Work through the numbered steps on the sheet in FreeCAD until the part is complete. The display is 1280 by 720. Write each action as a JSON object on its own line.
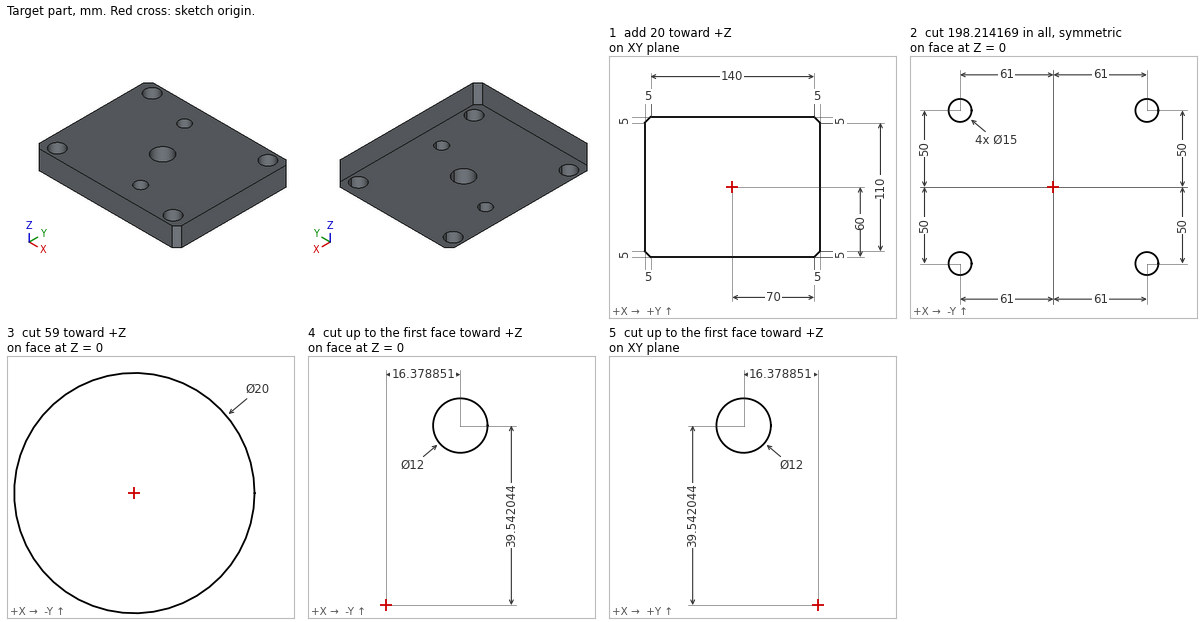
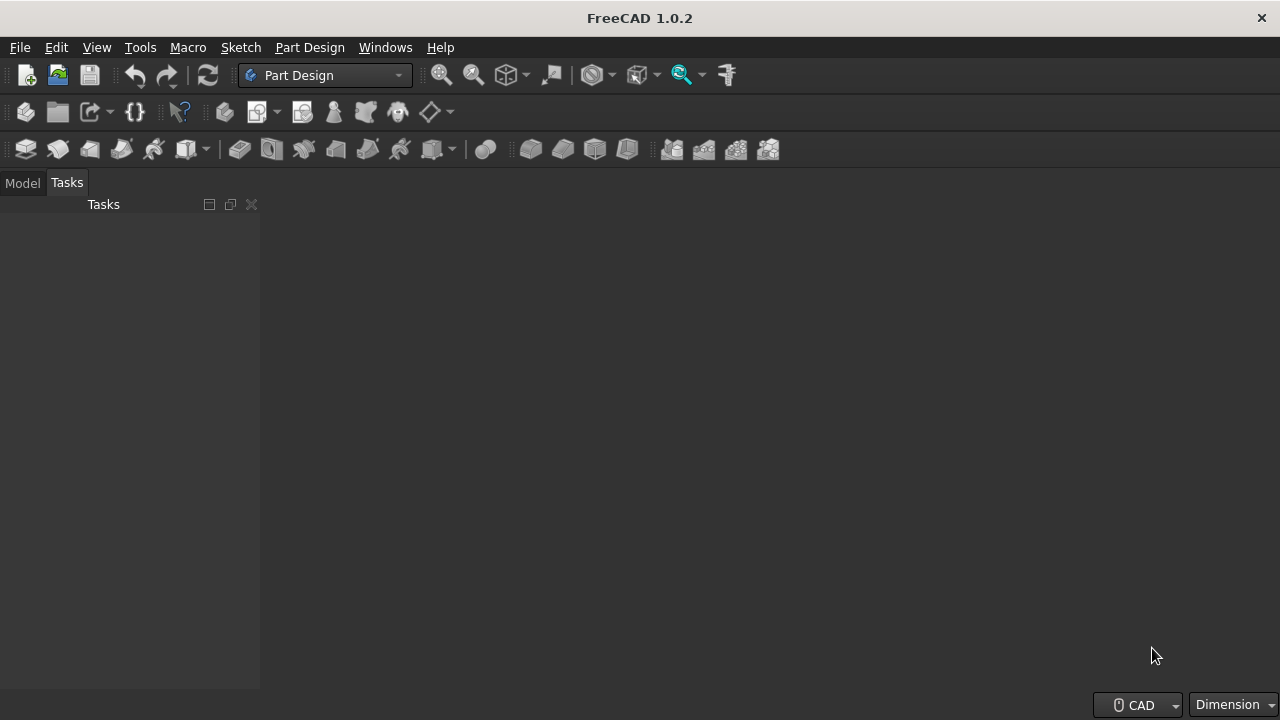
{"action": "key", "text": "ctrl+n"}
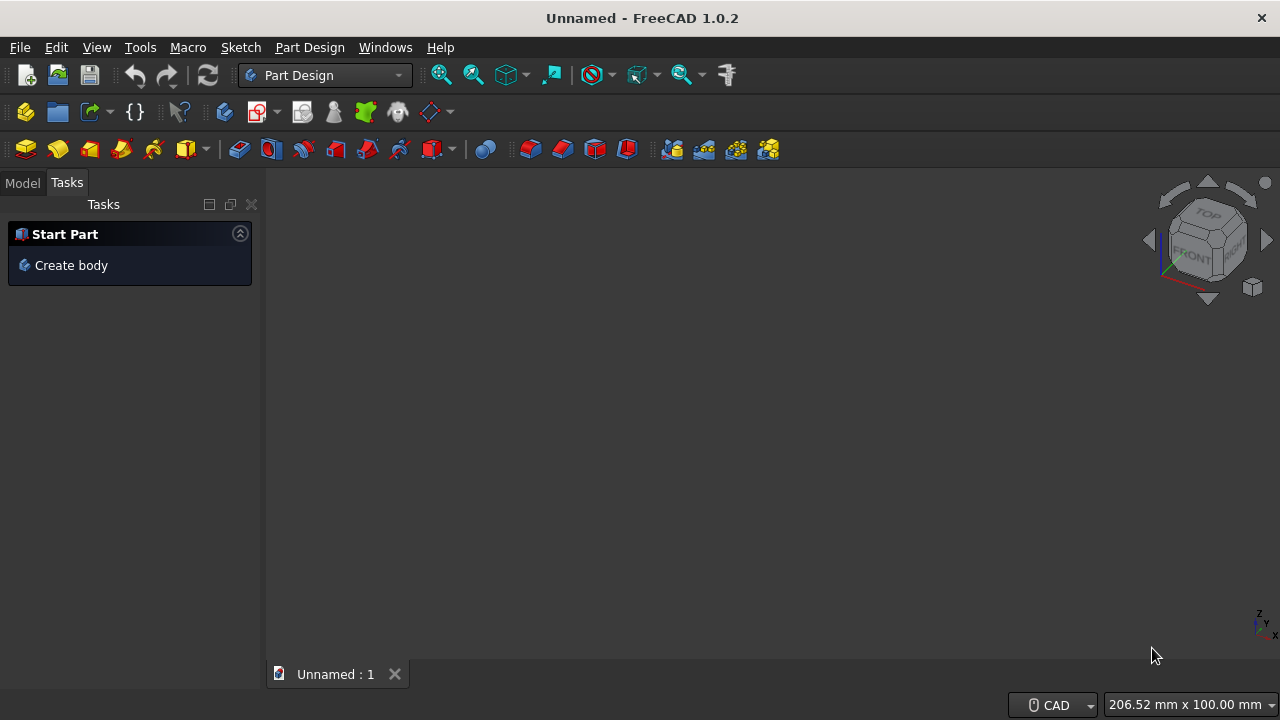
{"action": "left_click", "coordinate": [258, 112]}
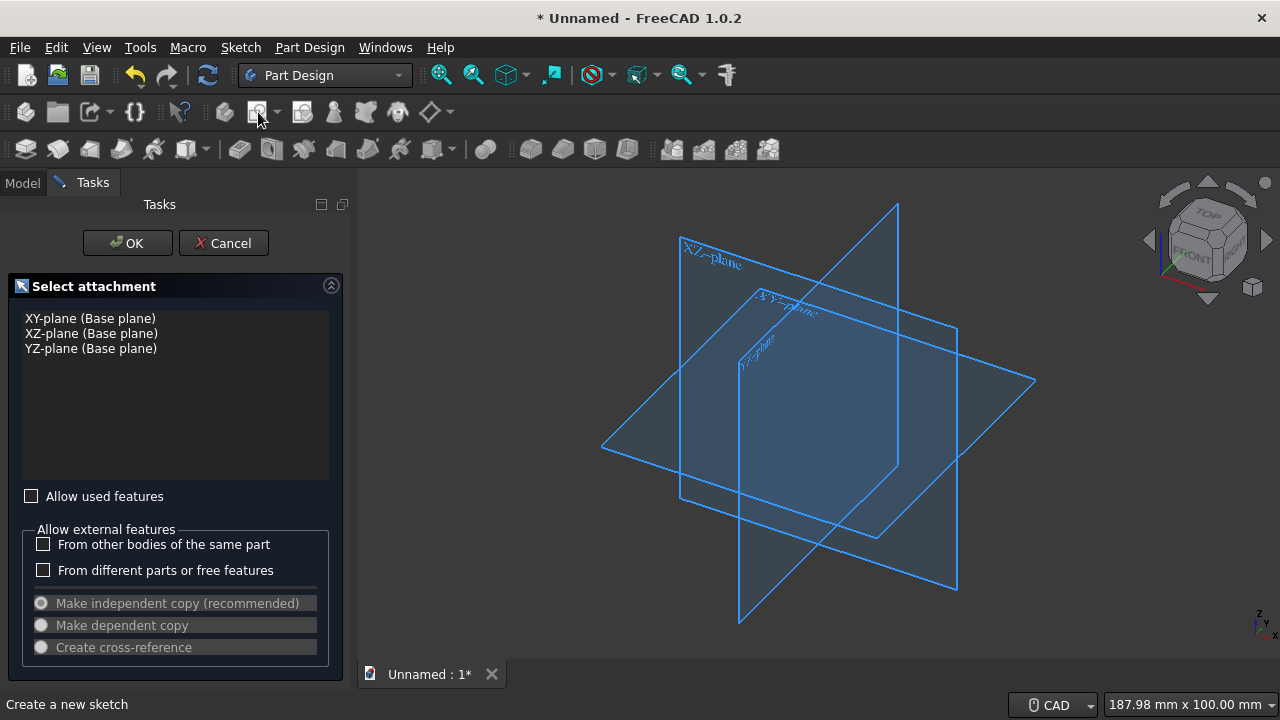
{"action": "left_click", "coordinate": [82, 318]}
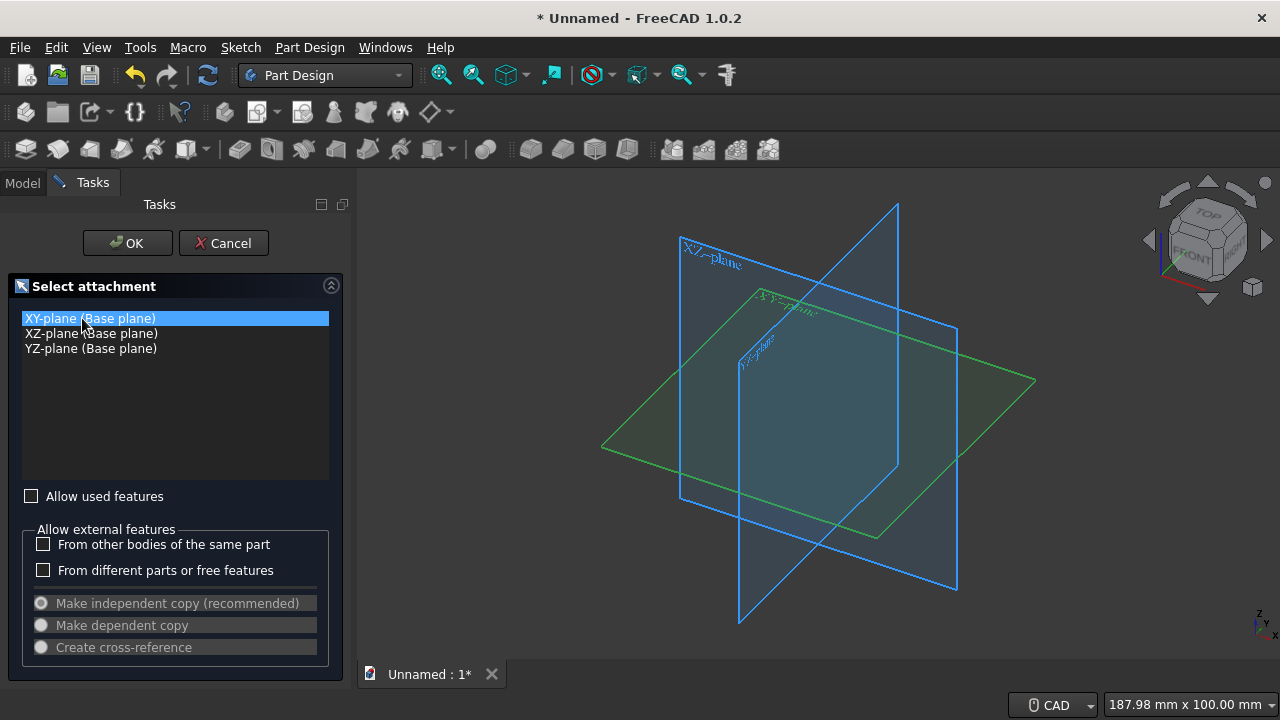
{"action": "left_click", "coordinate": [128, 243]}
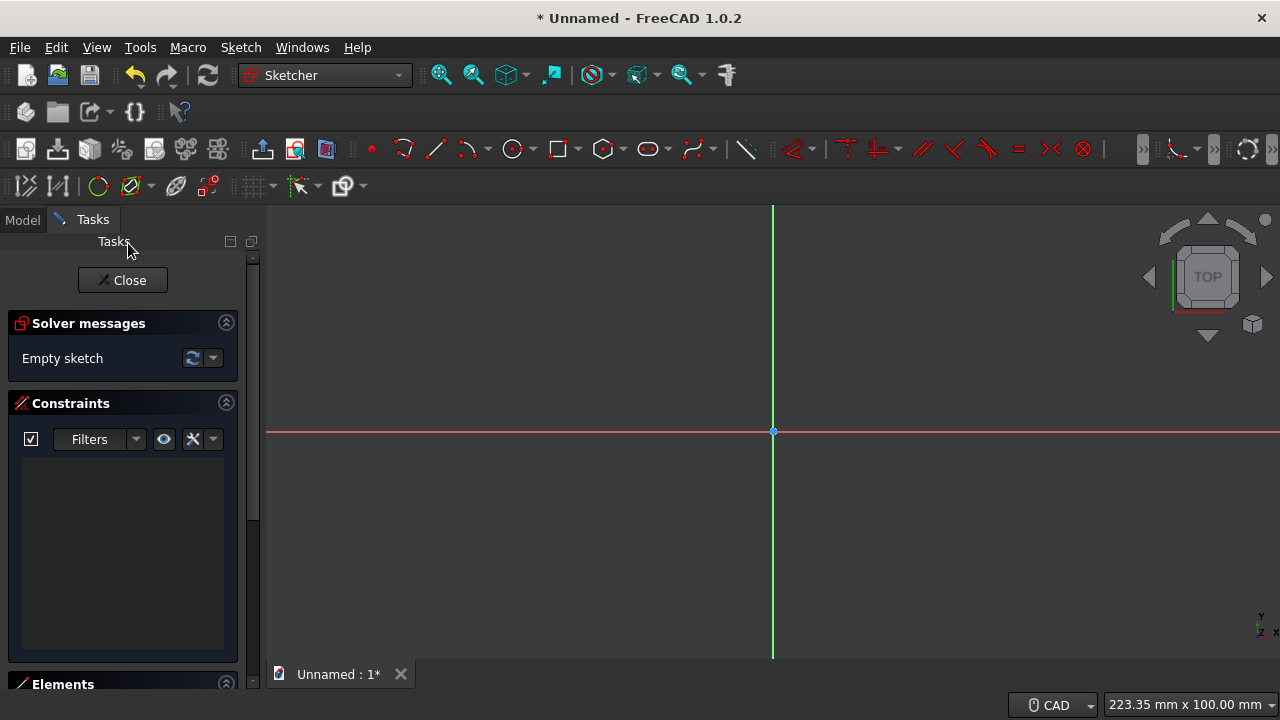
{"action": "scroll", "coordinate": [621, 432], "scroll_direction": "down", "scroll_amount": 3}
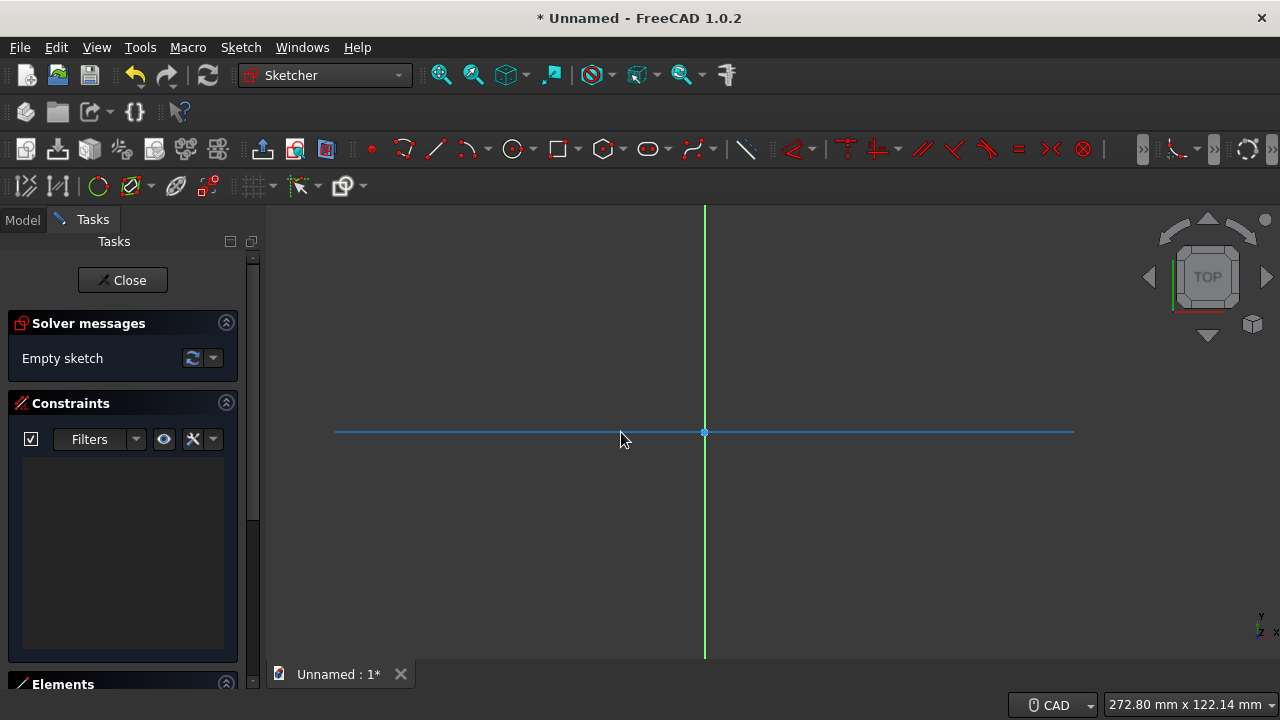
{"action": "left_click", "coordinate": [404, 150]}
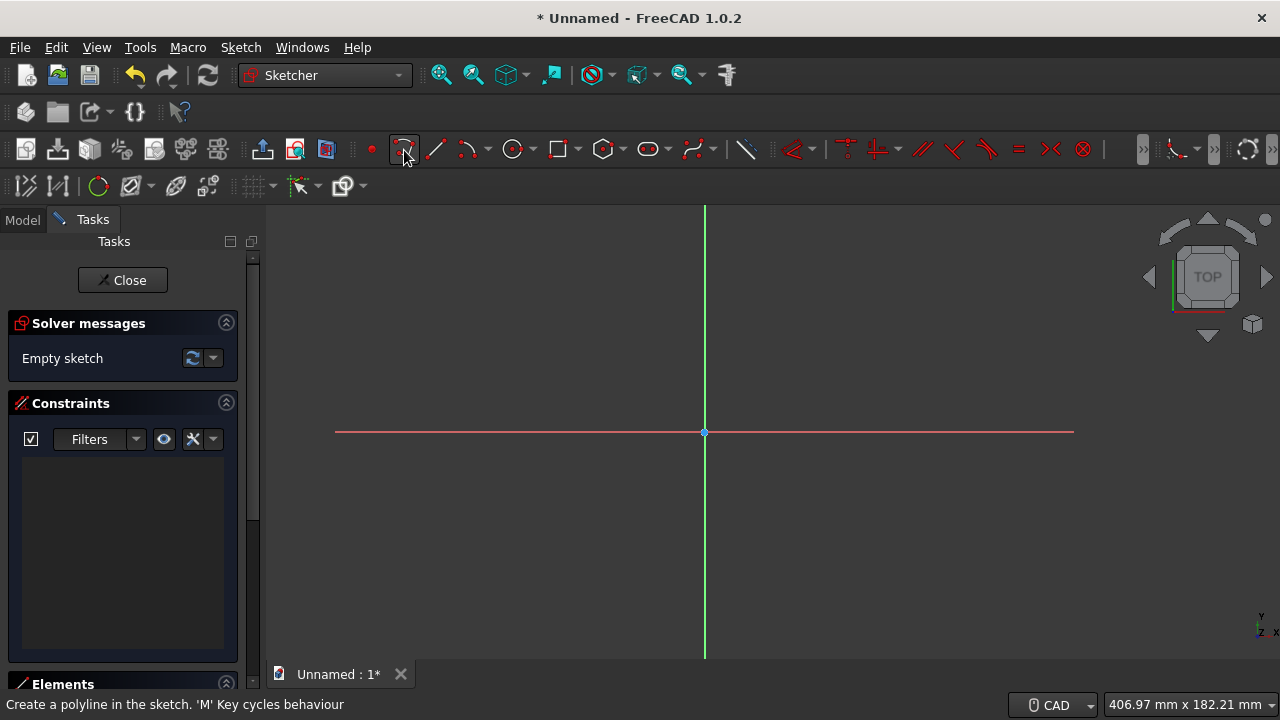
{"action": "left_click", "coordinate": [879, 582]}
{"action": "left_click", "coordinate": [891, 569]}
{"action": "left_click", "coordinate": [891, 295]}
{"action": "left_click", "coordinate": [879, 283]}
{"action": "left_click", "coordinate": [530, 283]}
{"action": "left_click", "coordinate": [518, 295]}
{"action": "left_click", "coordinate": [518, 569]}
{"action": "left_click", "coordinate": [530, 582]}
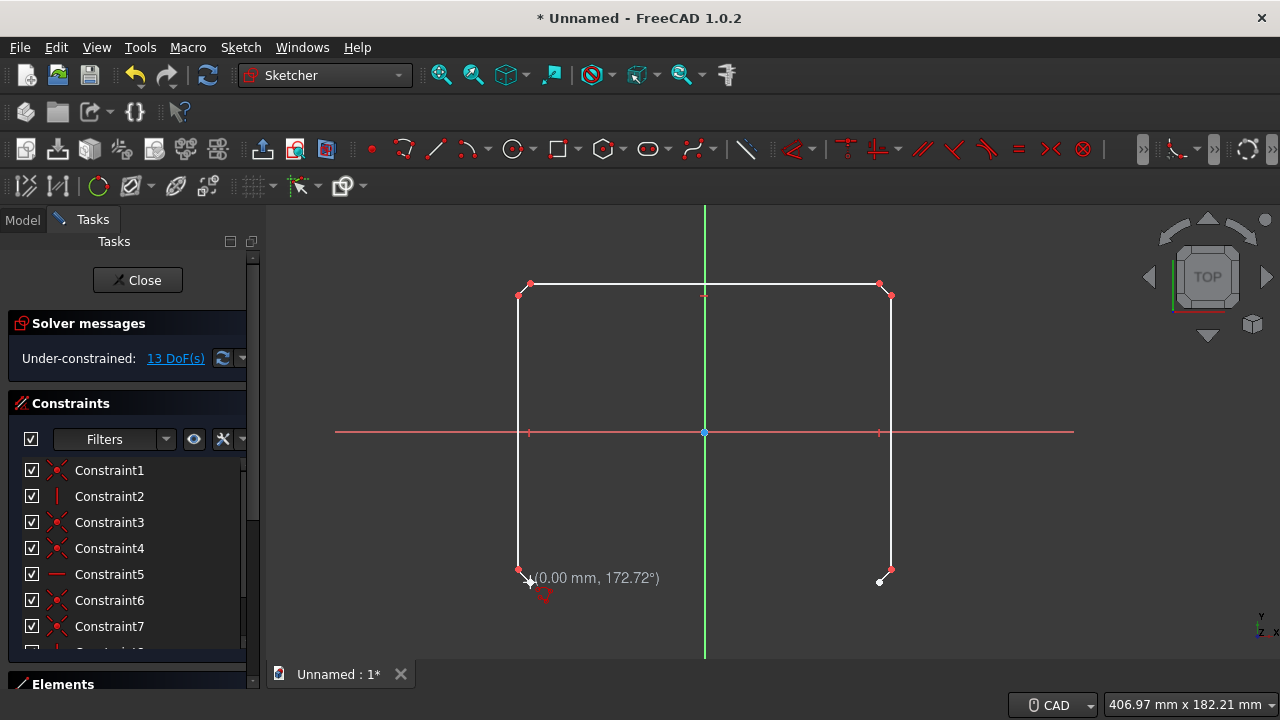
{"action": "scroll", "coordinate": [879, 582], "scroll_direction": "up", "scroll_amount": 3}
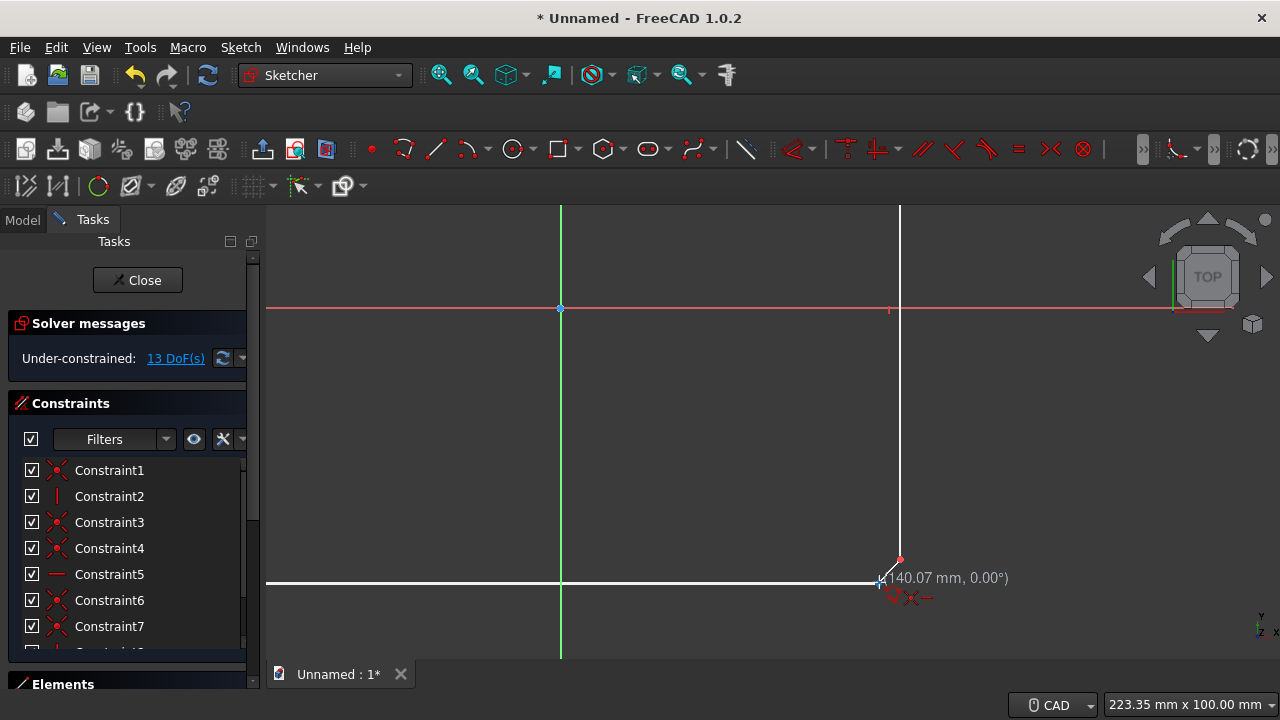
{"action": "left_click", "coordinate": [879, 583]}
{"action": "key", "text": "Escape"}
{"action": "key", "text": "Escape"}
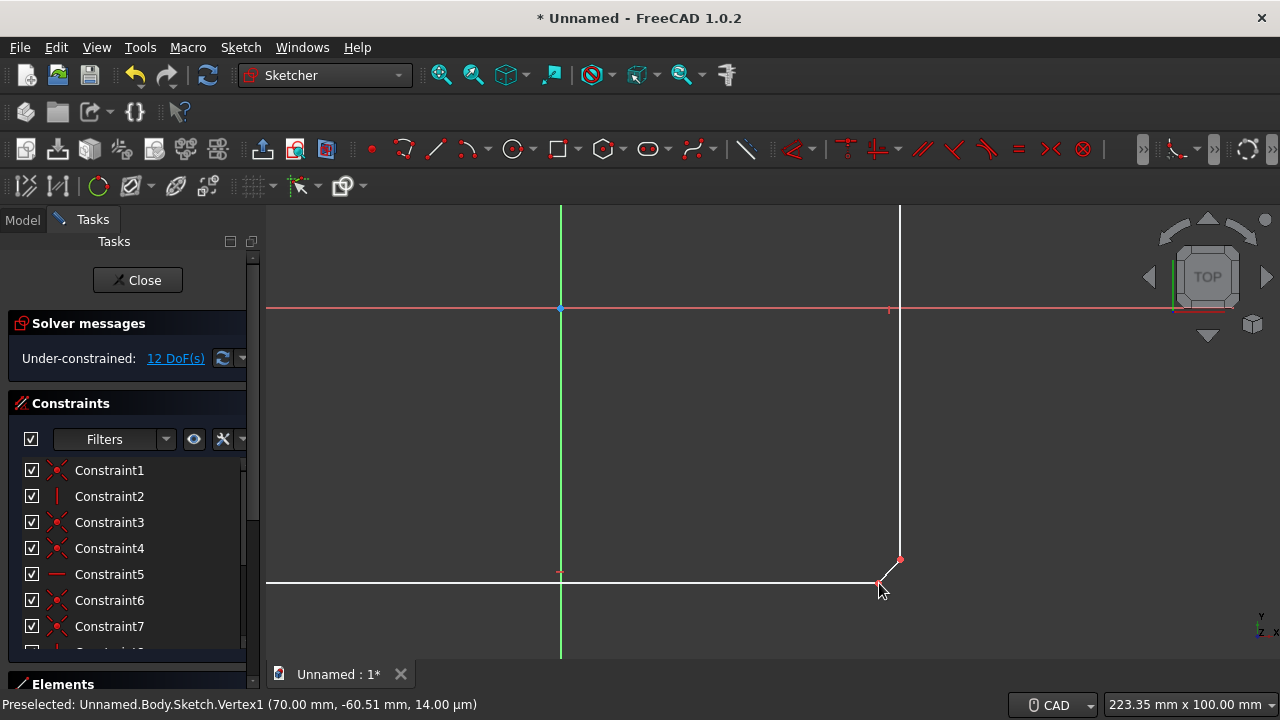
{"action": "scroll", "coordinate": [885, 576], "scroll_direction": "up", "scroll_amount": 3}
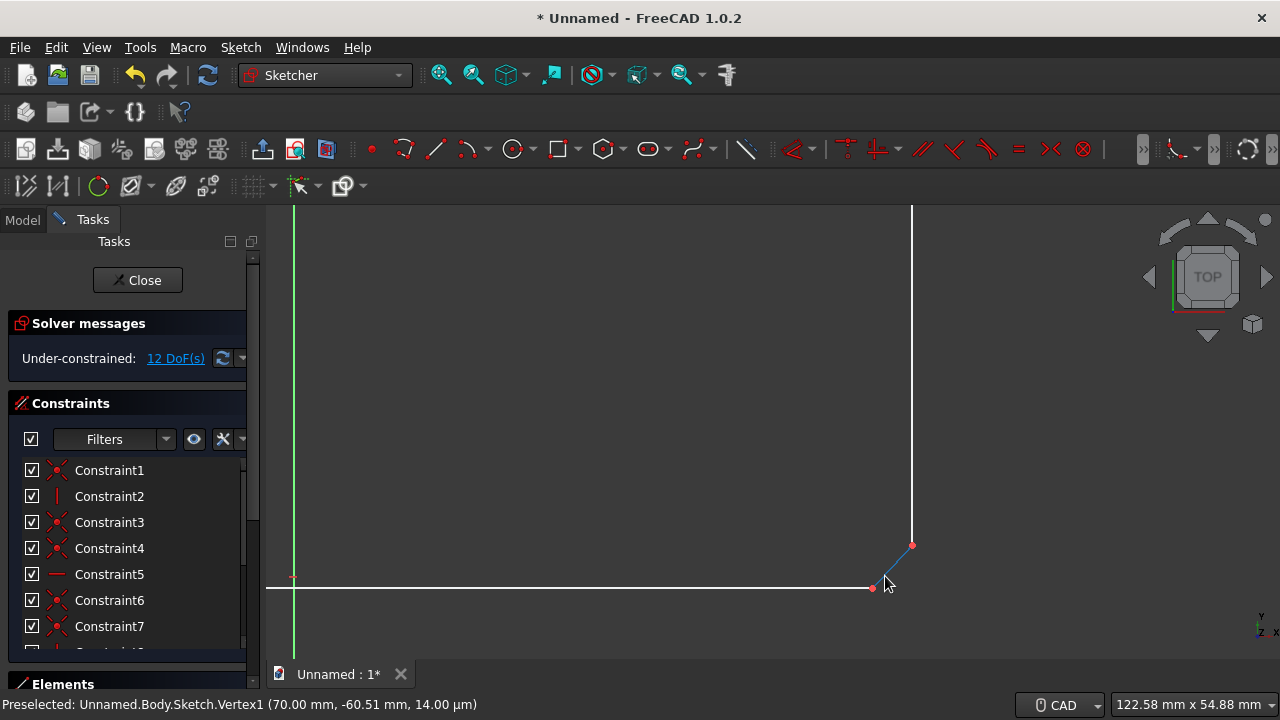
{"action": "left_click", "coordinate": [885, 575]}